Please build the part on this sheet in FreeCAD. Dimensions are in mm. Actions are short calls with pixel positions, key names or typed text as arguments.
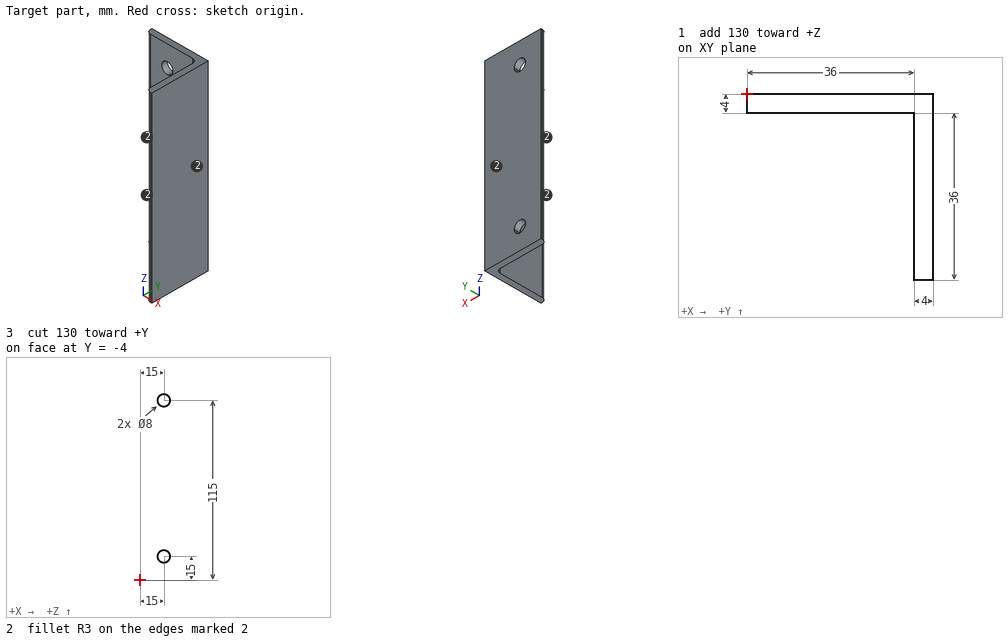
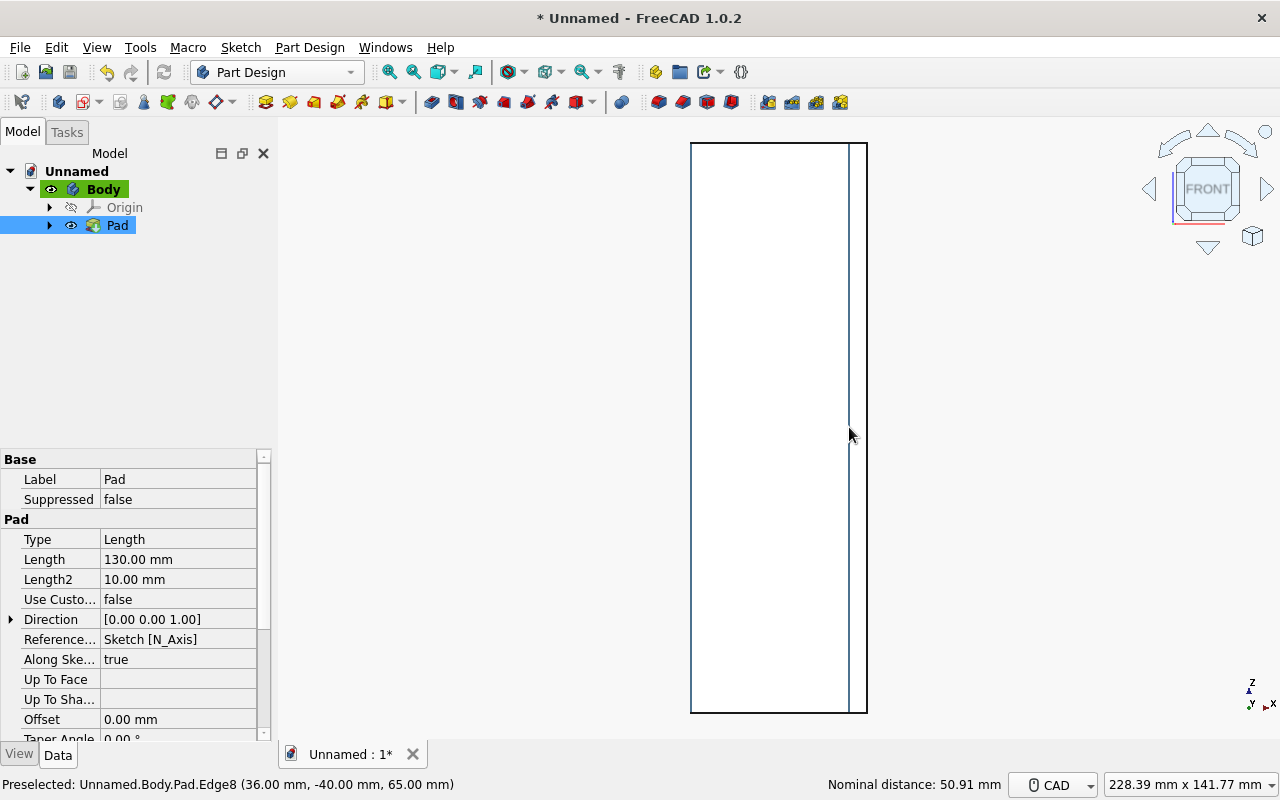
key(3)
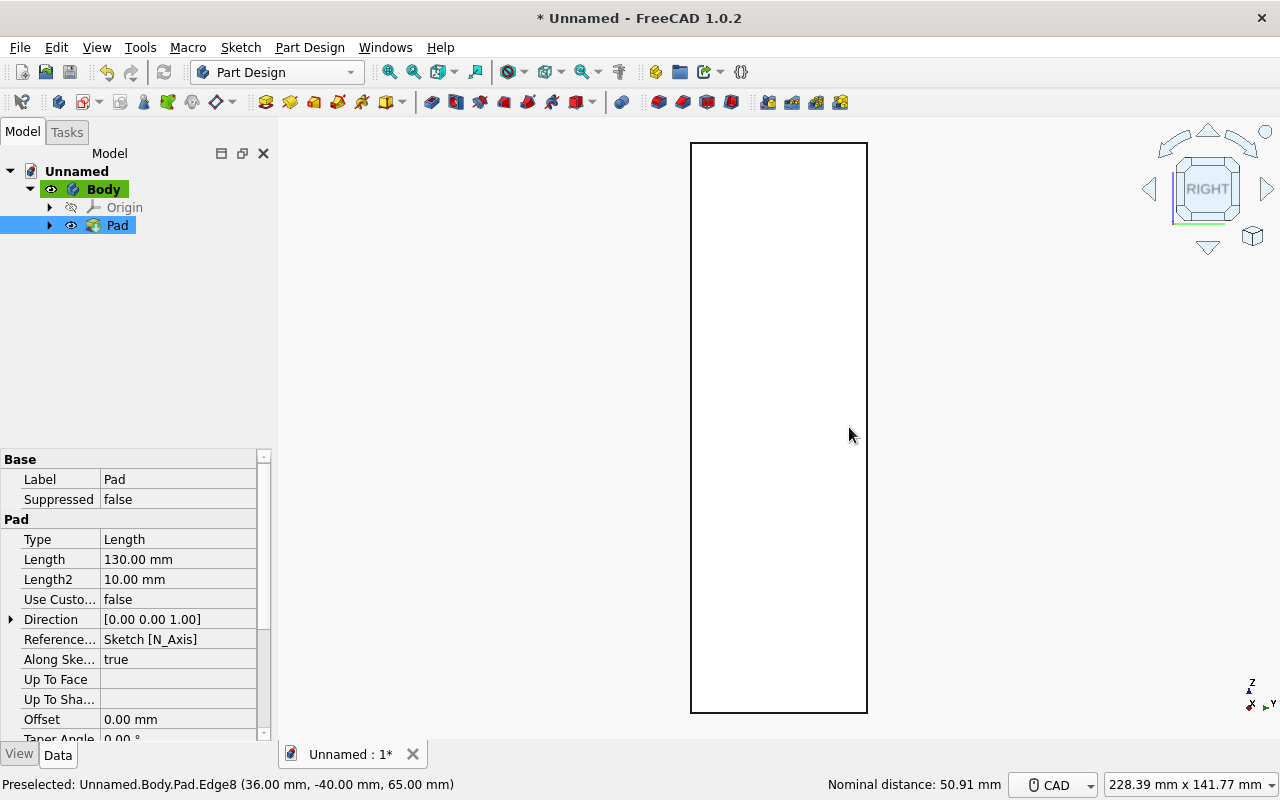
key(5)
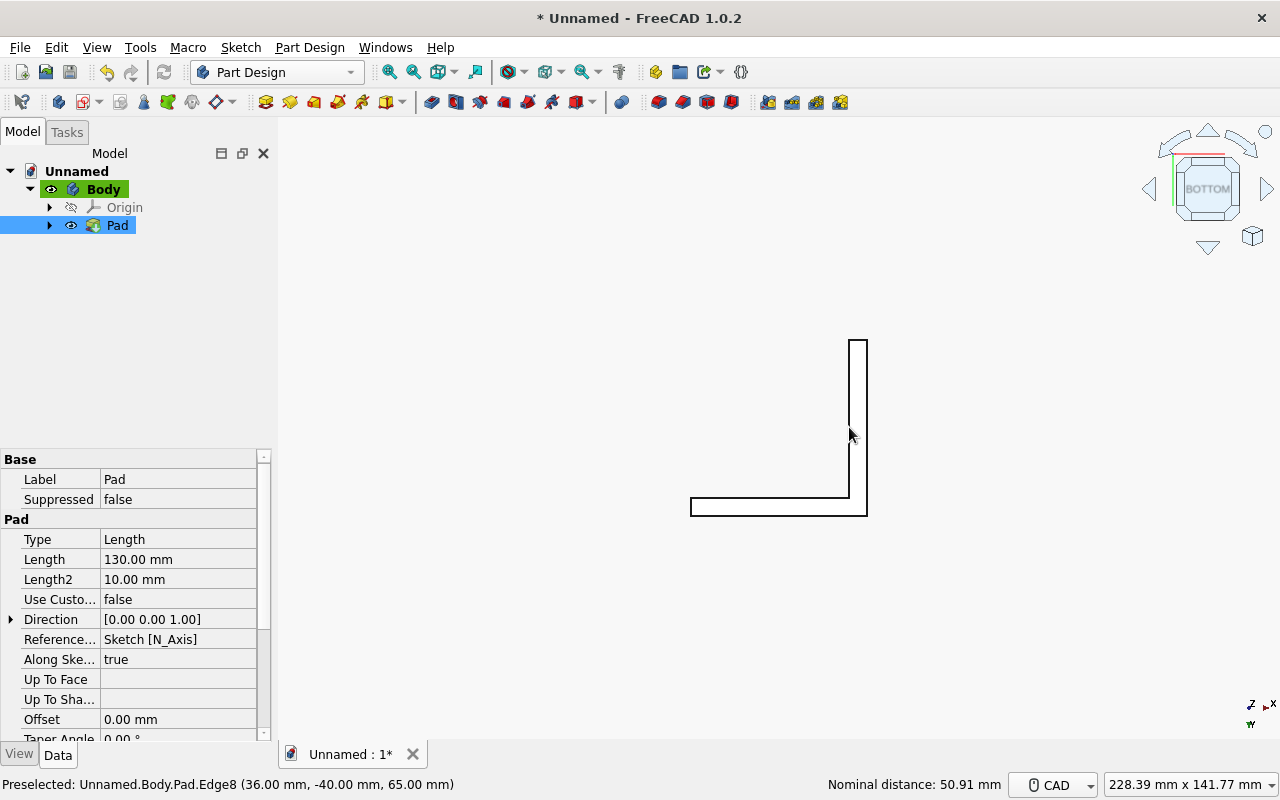
click(390, 72)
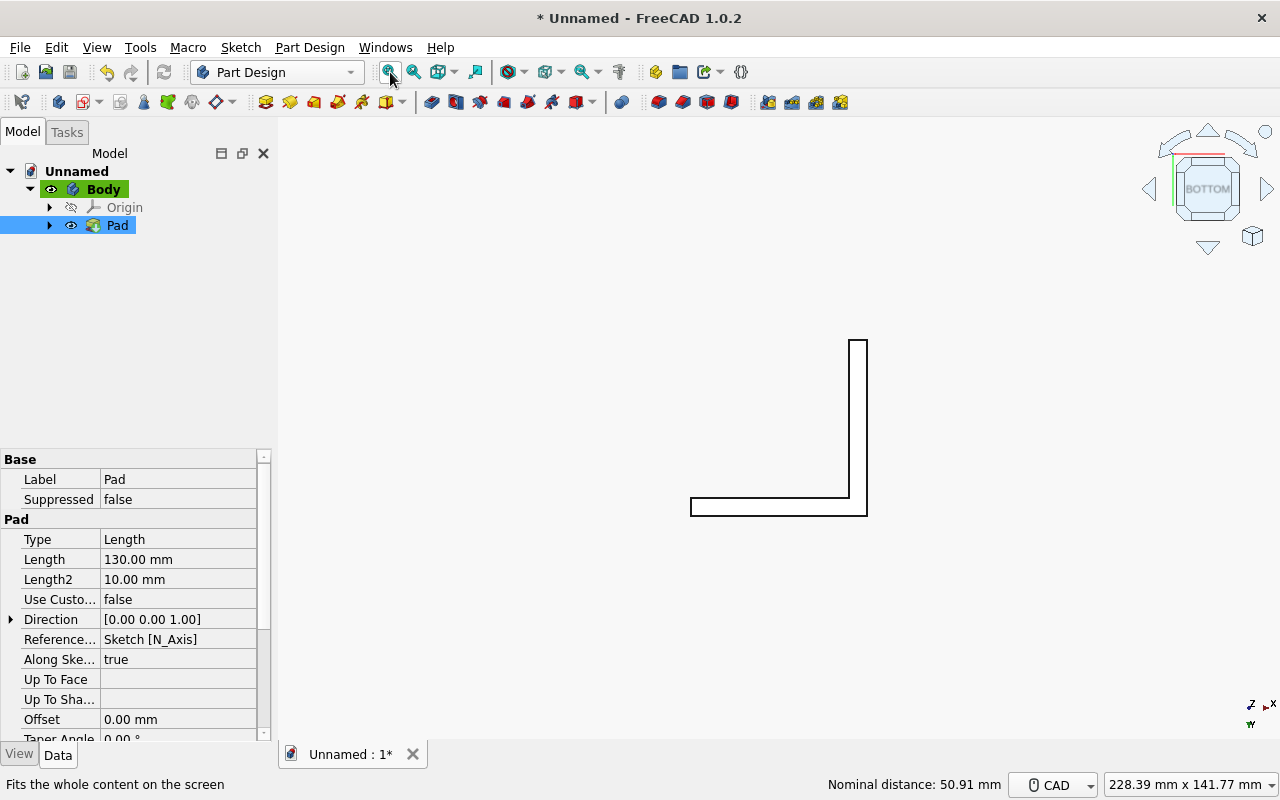
key(4)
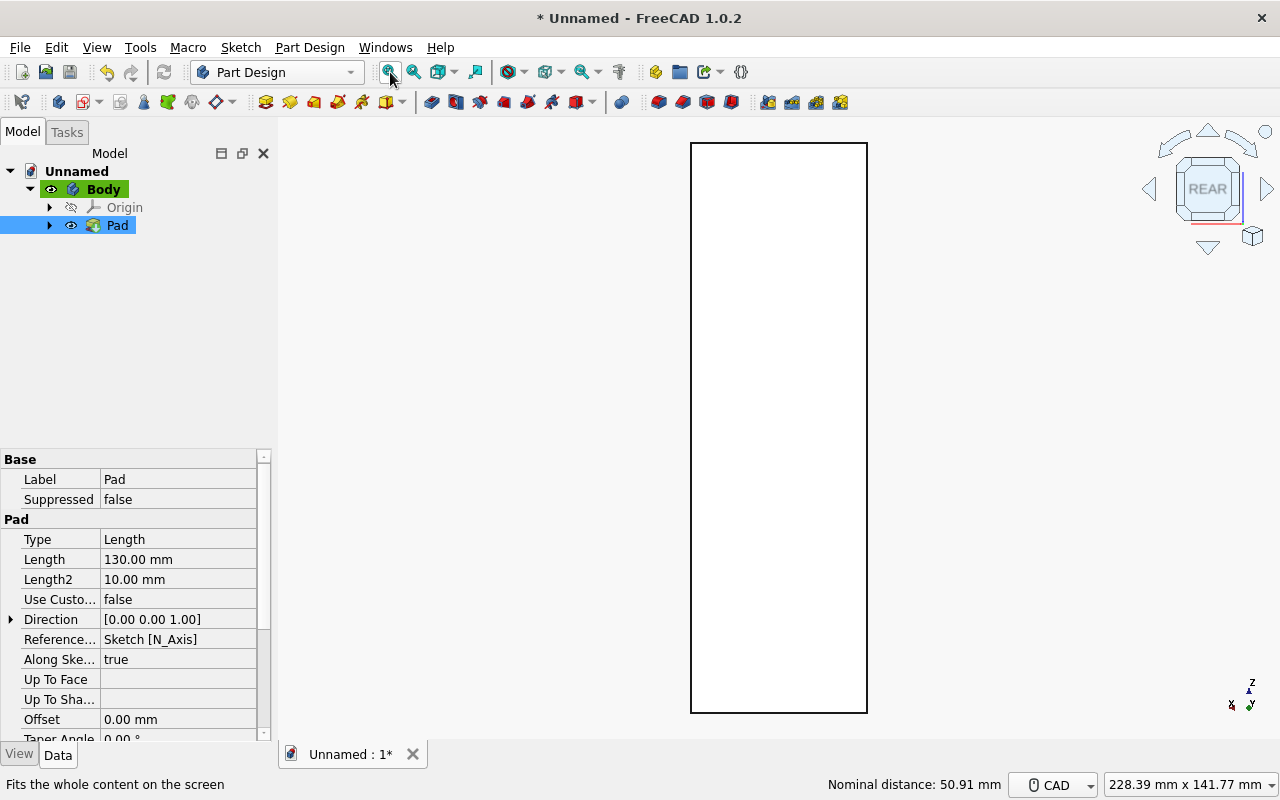
key(6)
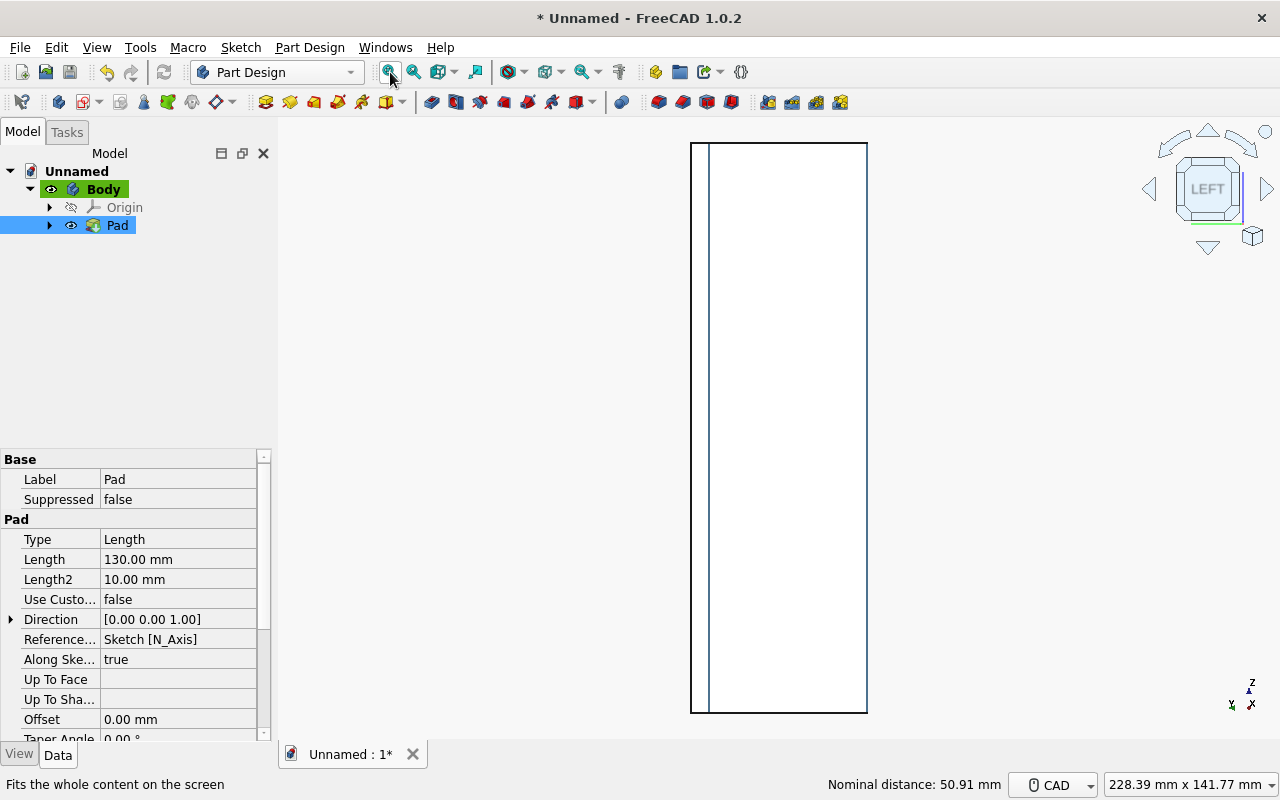
key(v)
key(3)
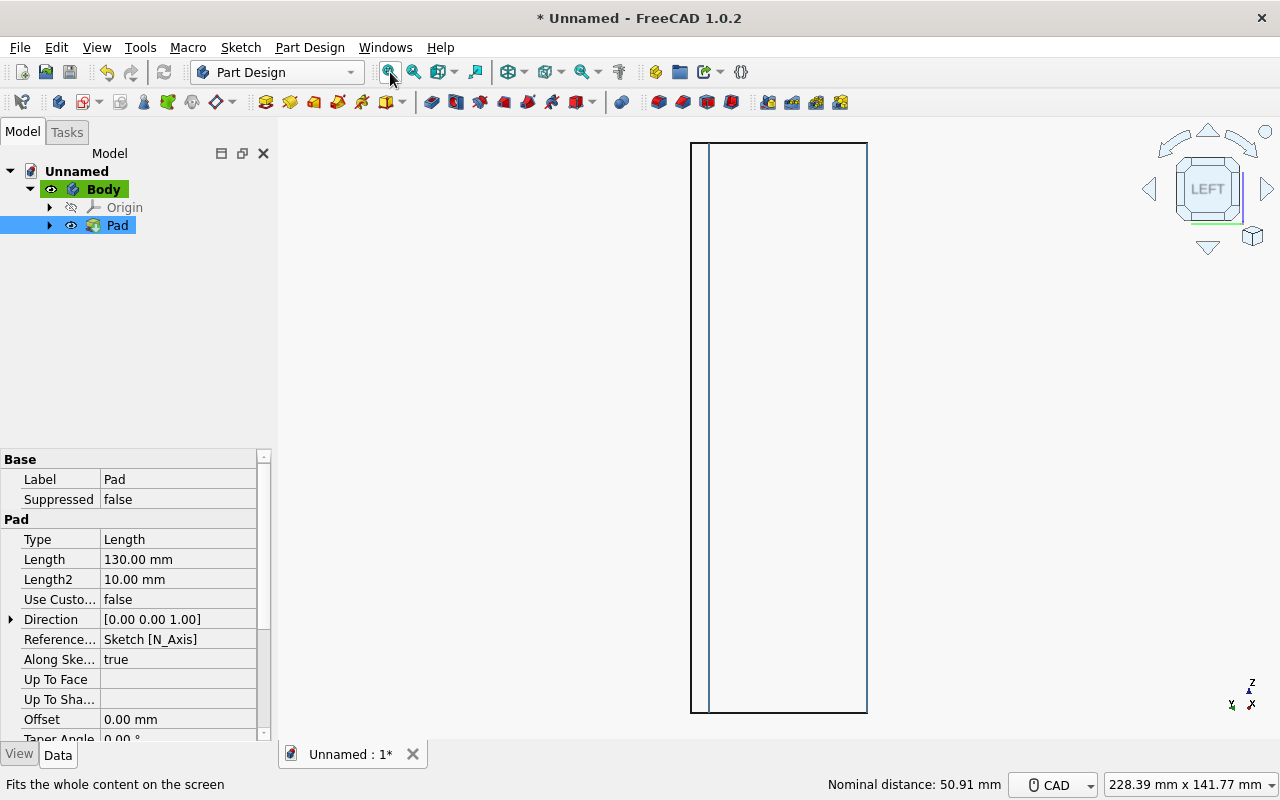
key(0)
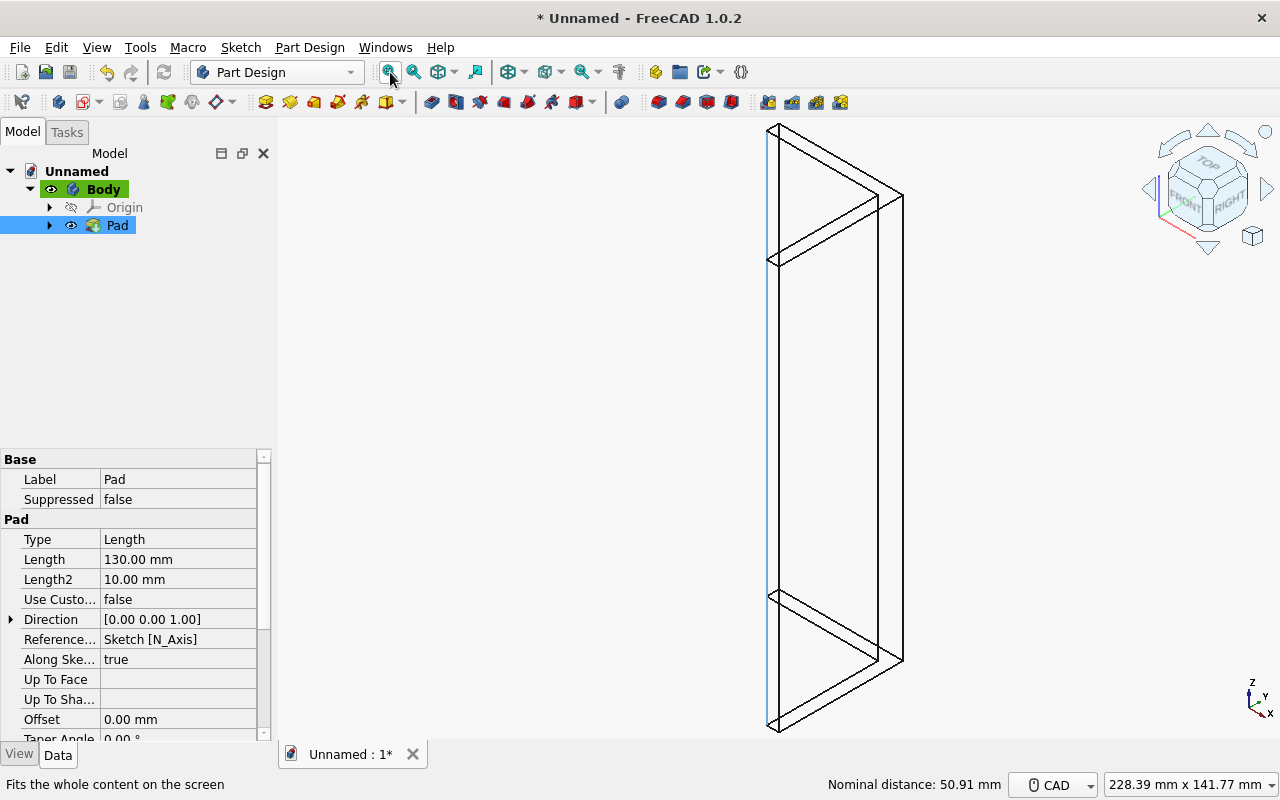
click(878, 427, ctrl)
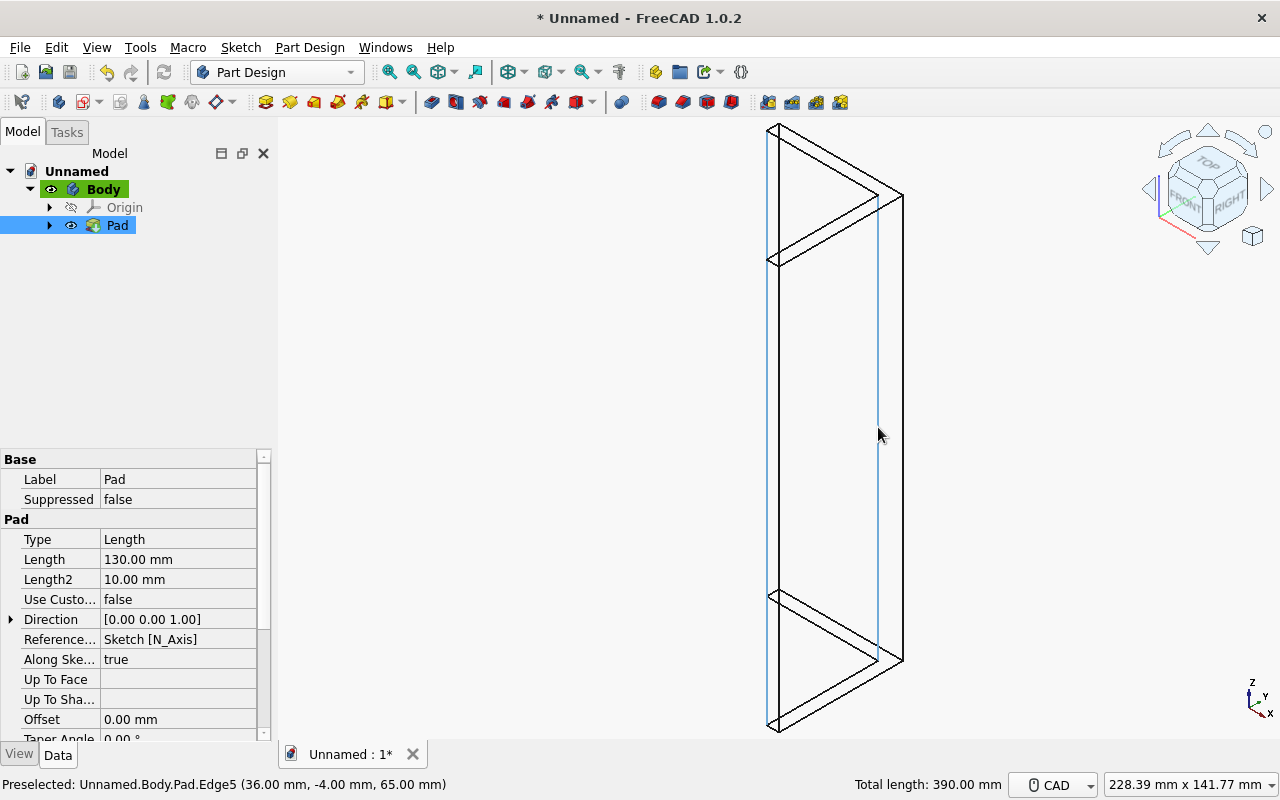
key(v)
key(1)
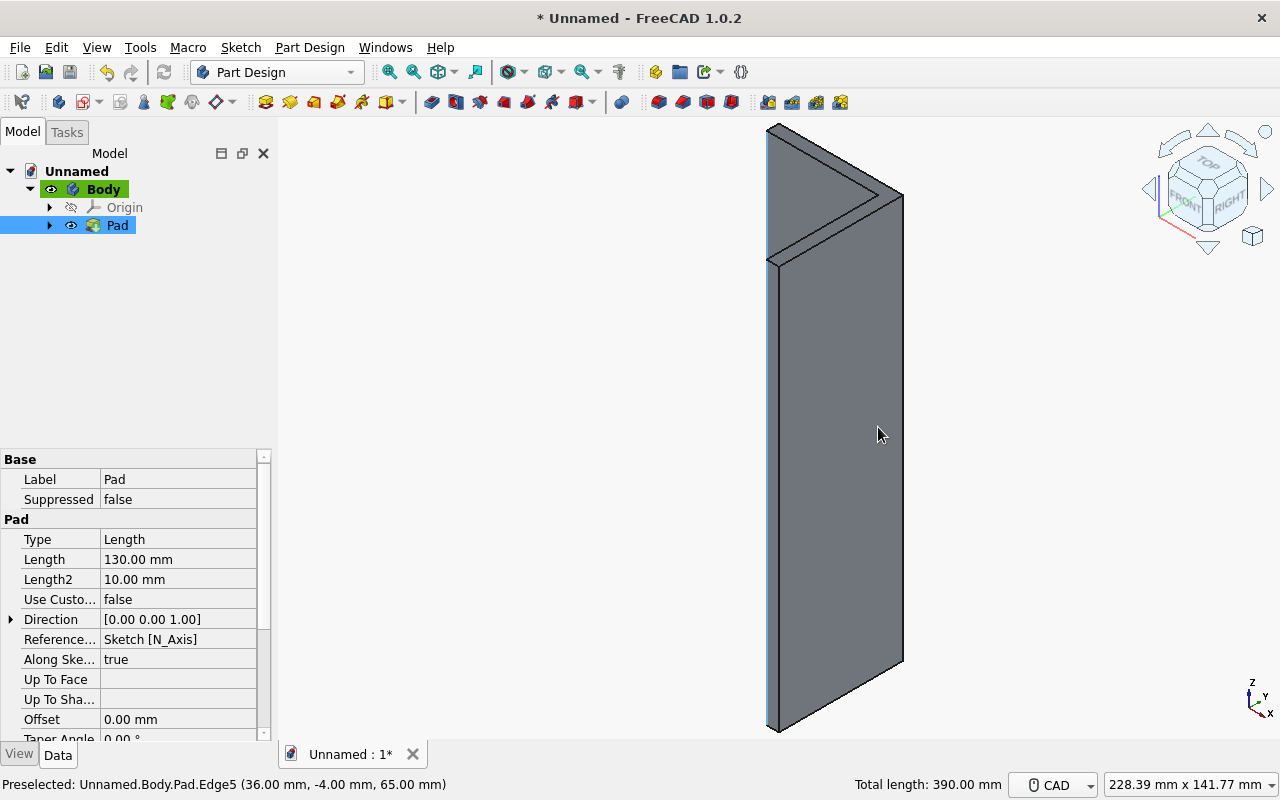
click(660, 102)